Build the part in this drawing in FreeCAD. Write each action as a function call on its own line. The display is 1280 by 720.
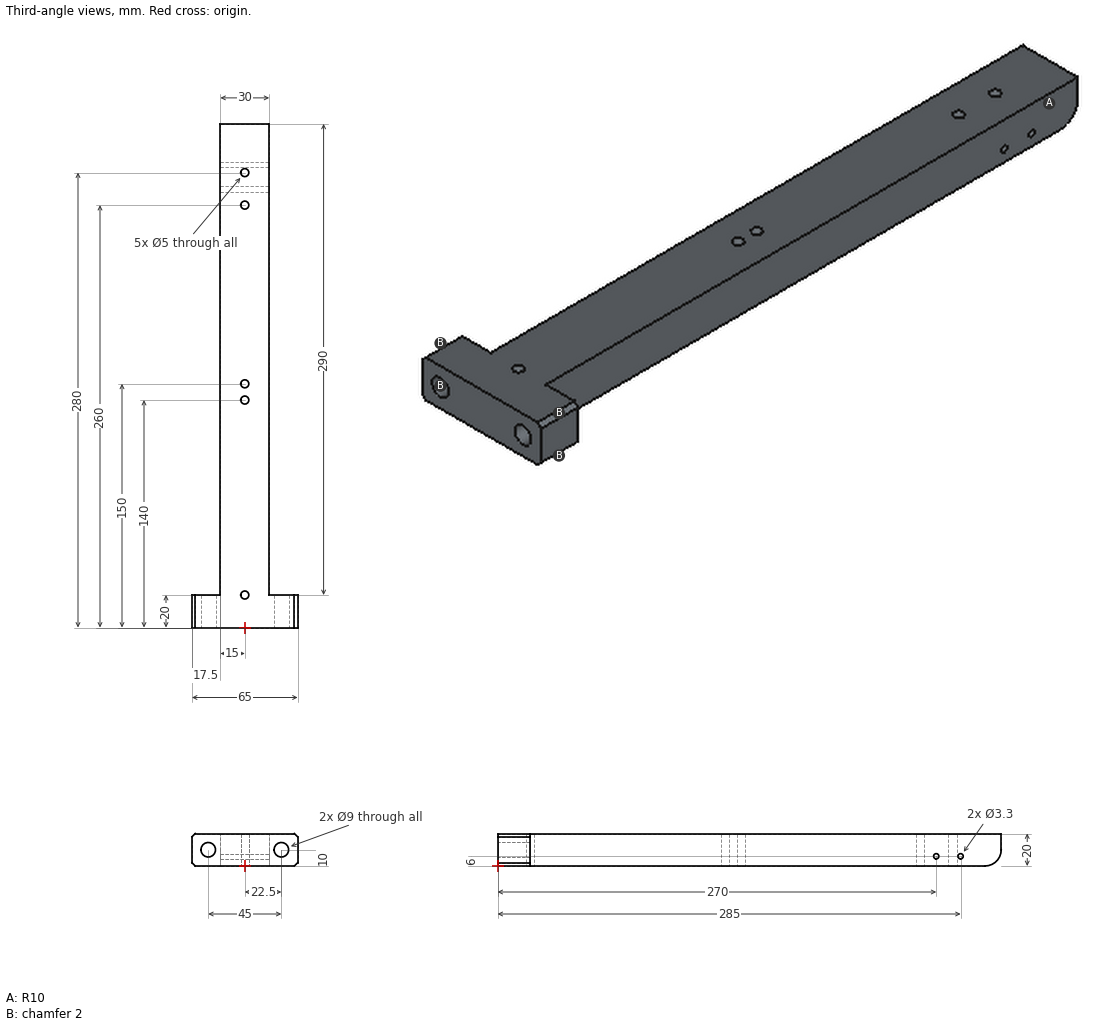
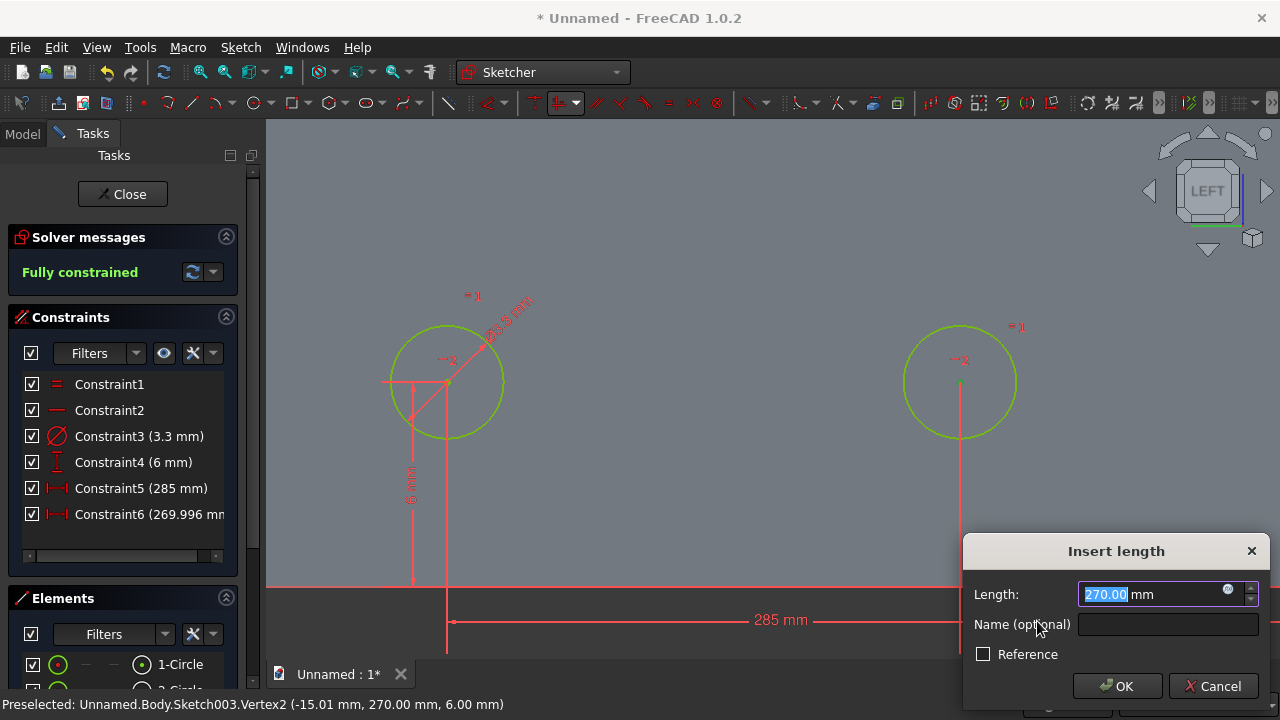
text(270)
key(Return)
key(Escape)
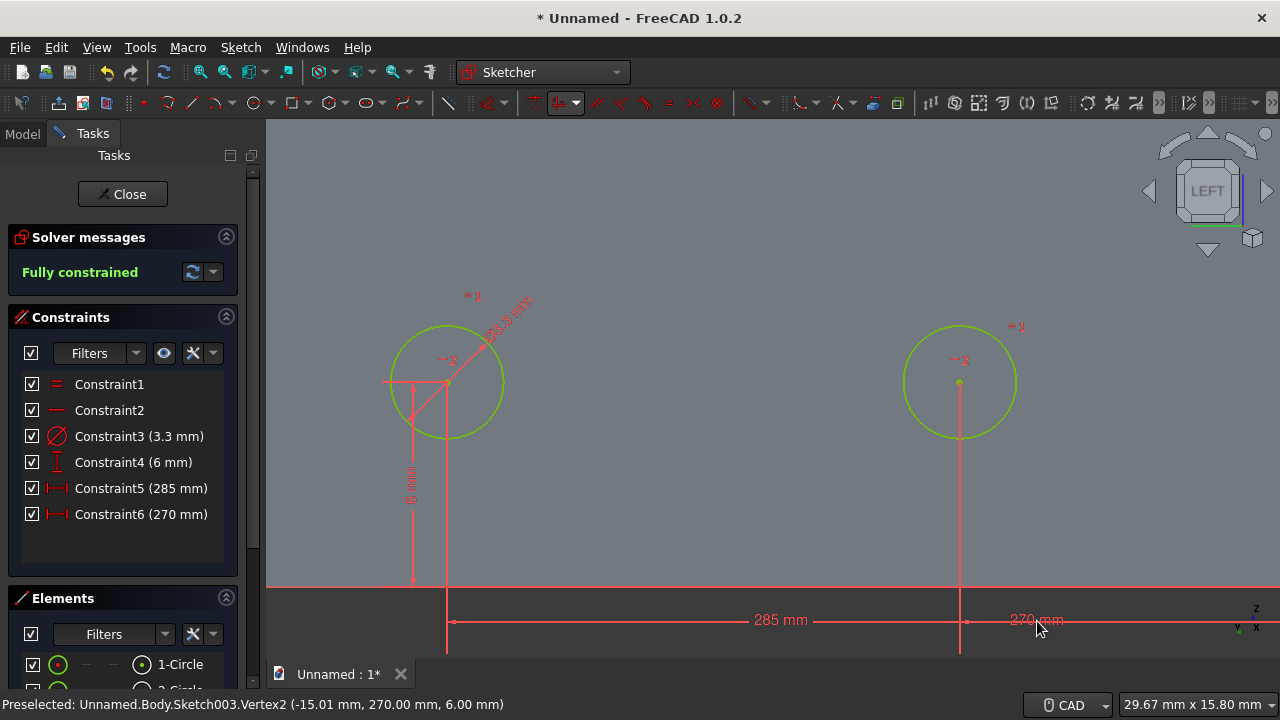
click(123, 194)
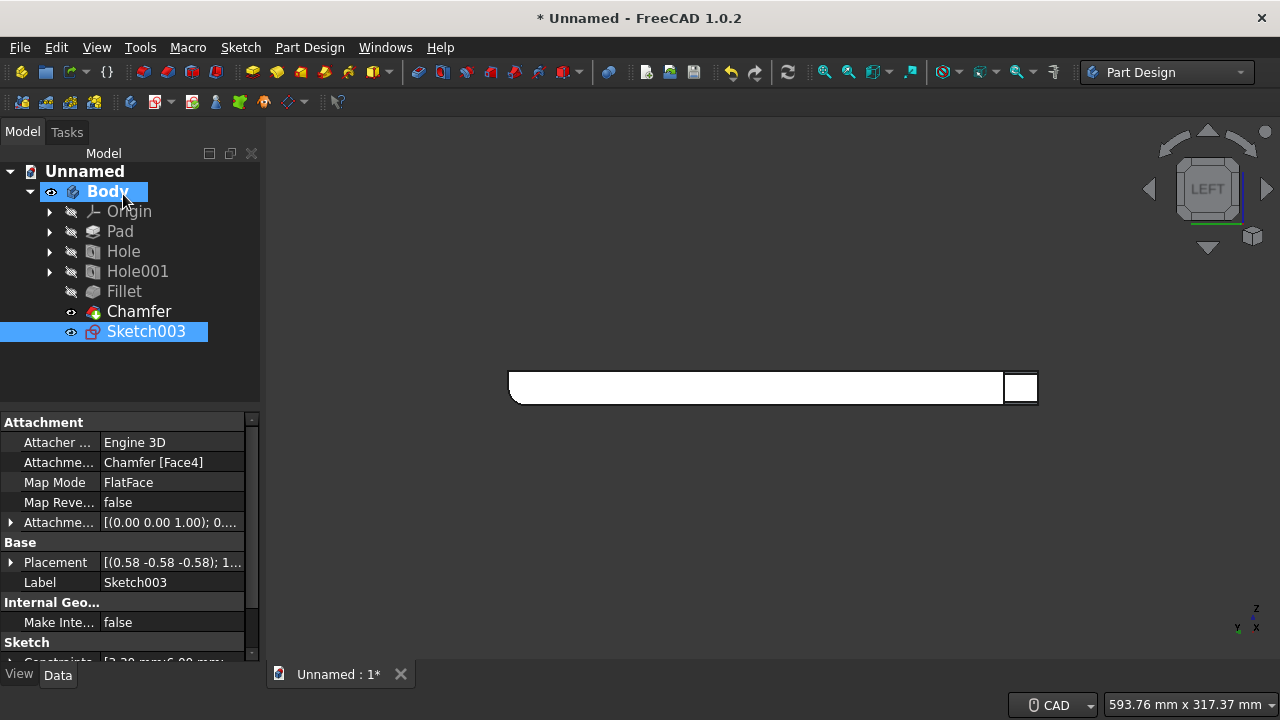
click(420, 72)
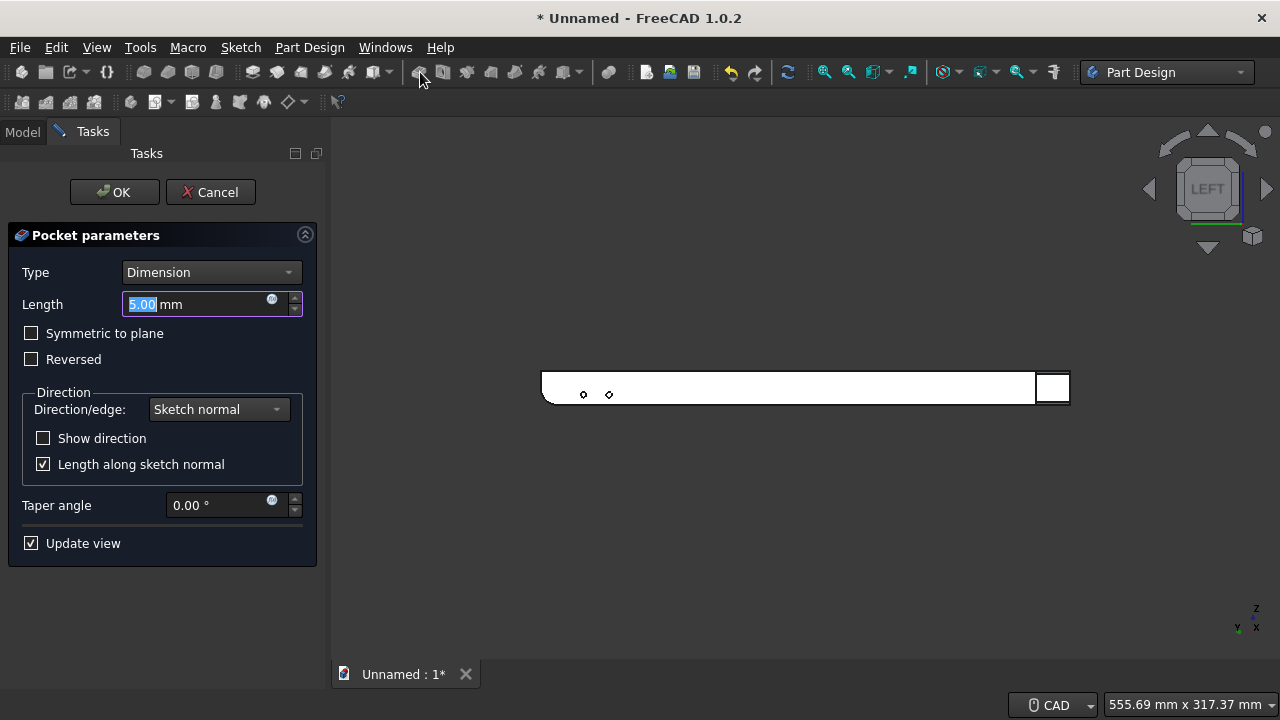
click(212, 272)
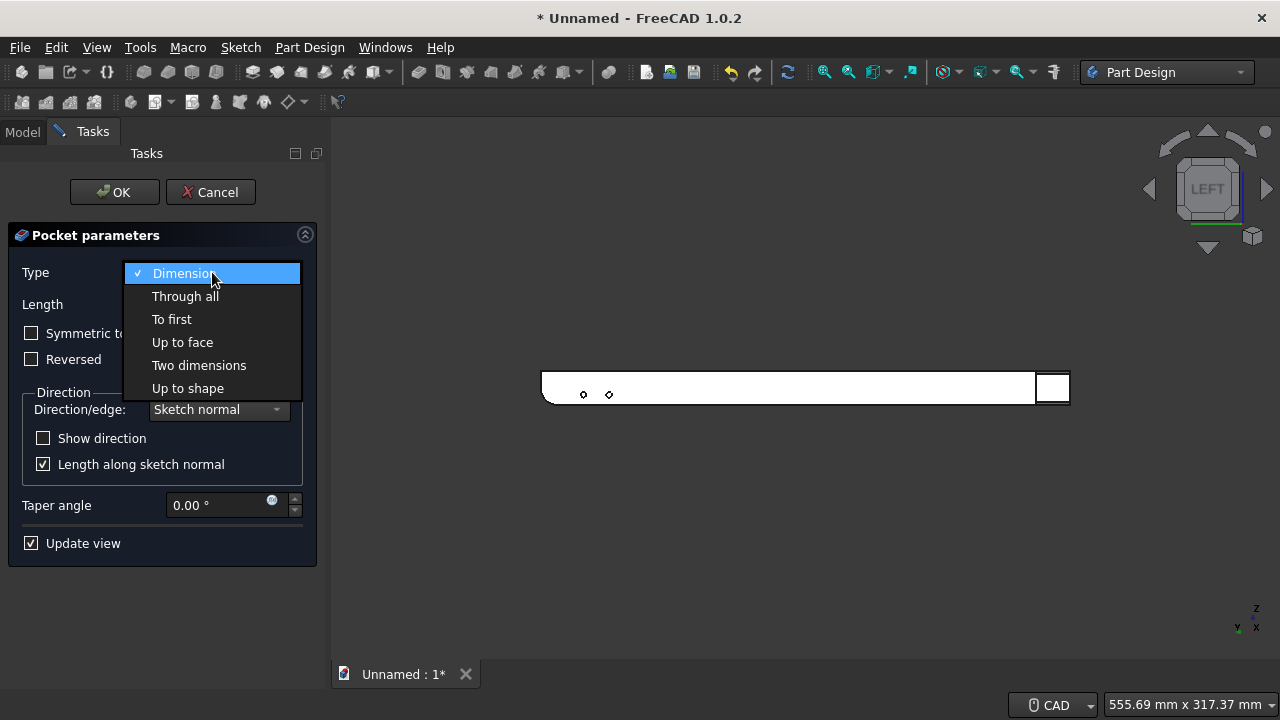
click(212, 296)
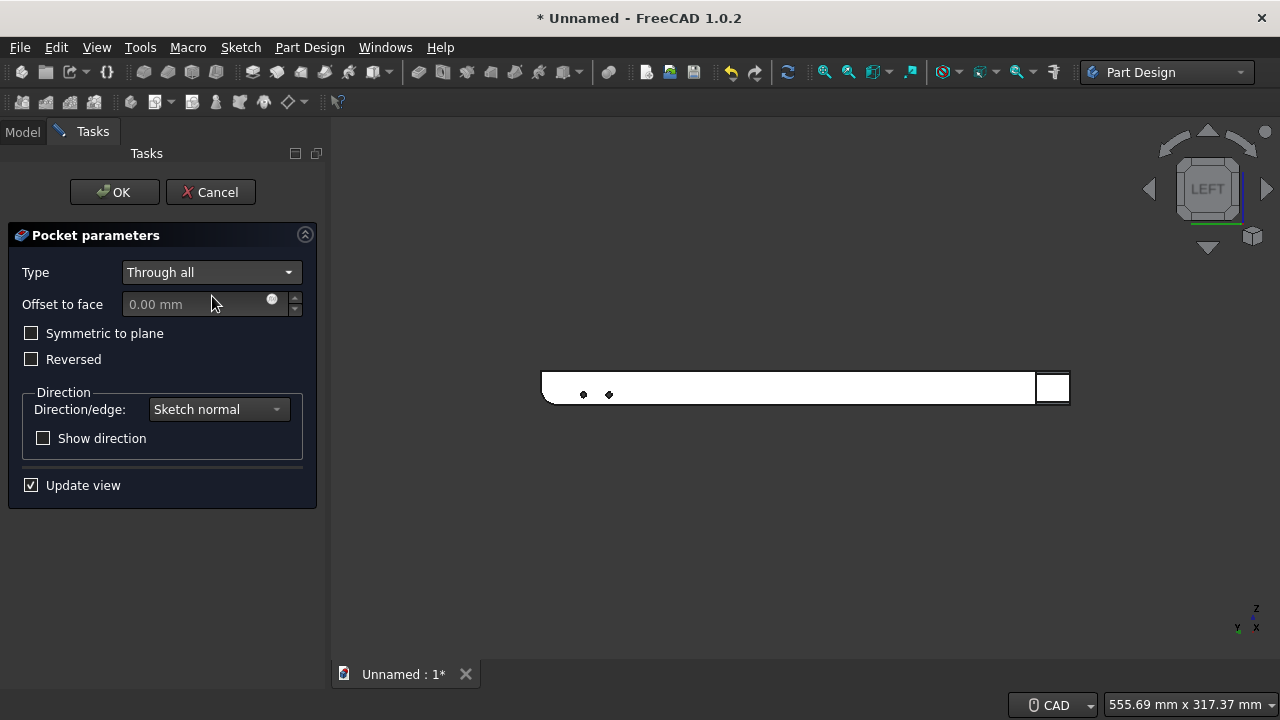
click(115, 192)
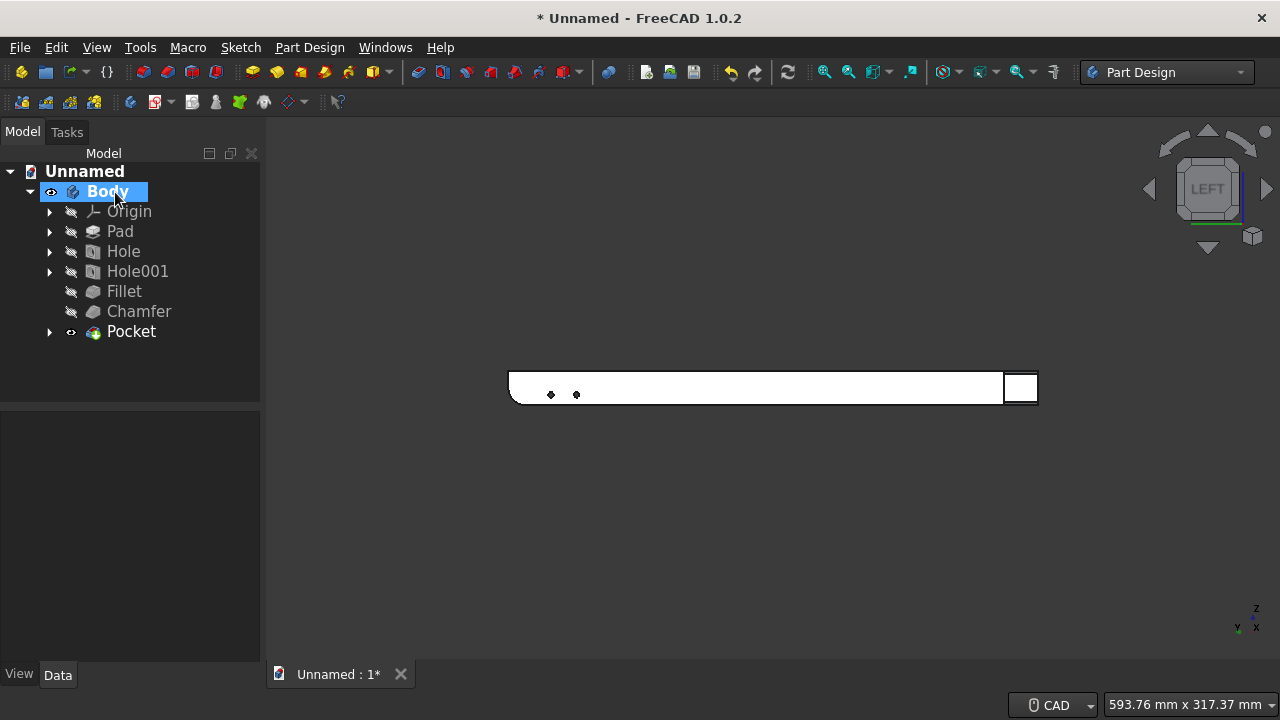
key(0)